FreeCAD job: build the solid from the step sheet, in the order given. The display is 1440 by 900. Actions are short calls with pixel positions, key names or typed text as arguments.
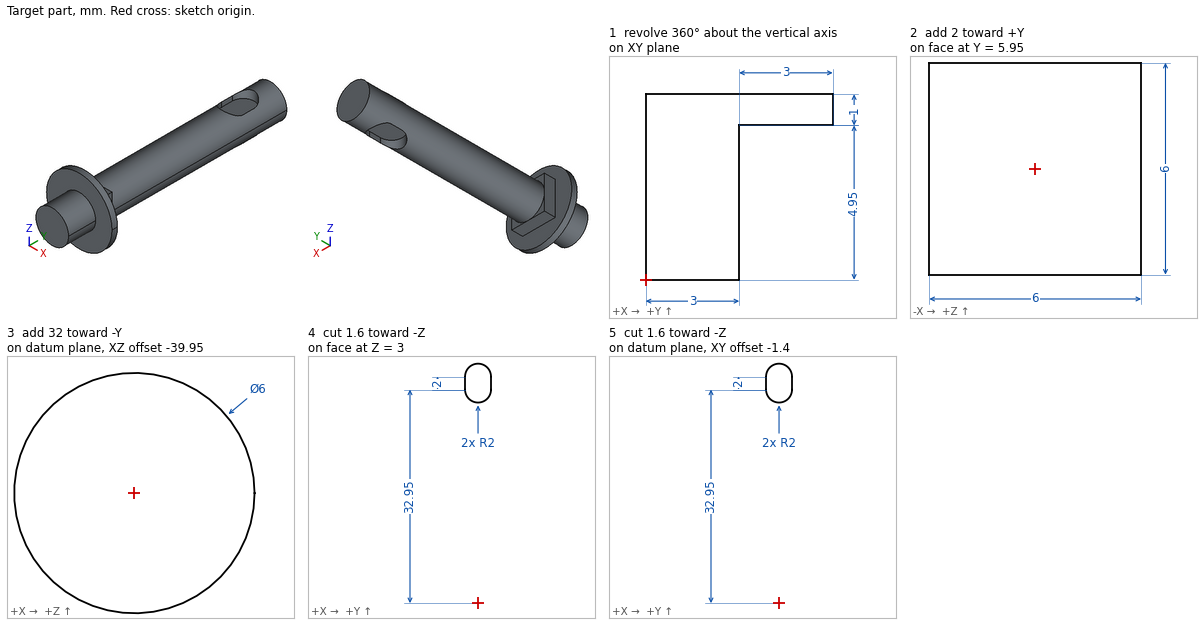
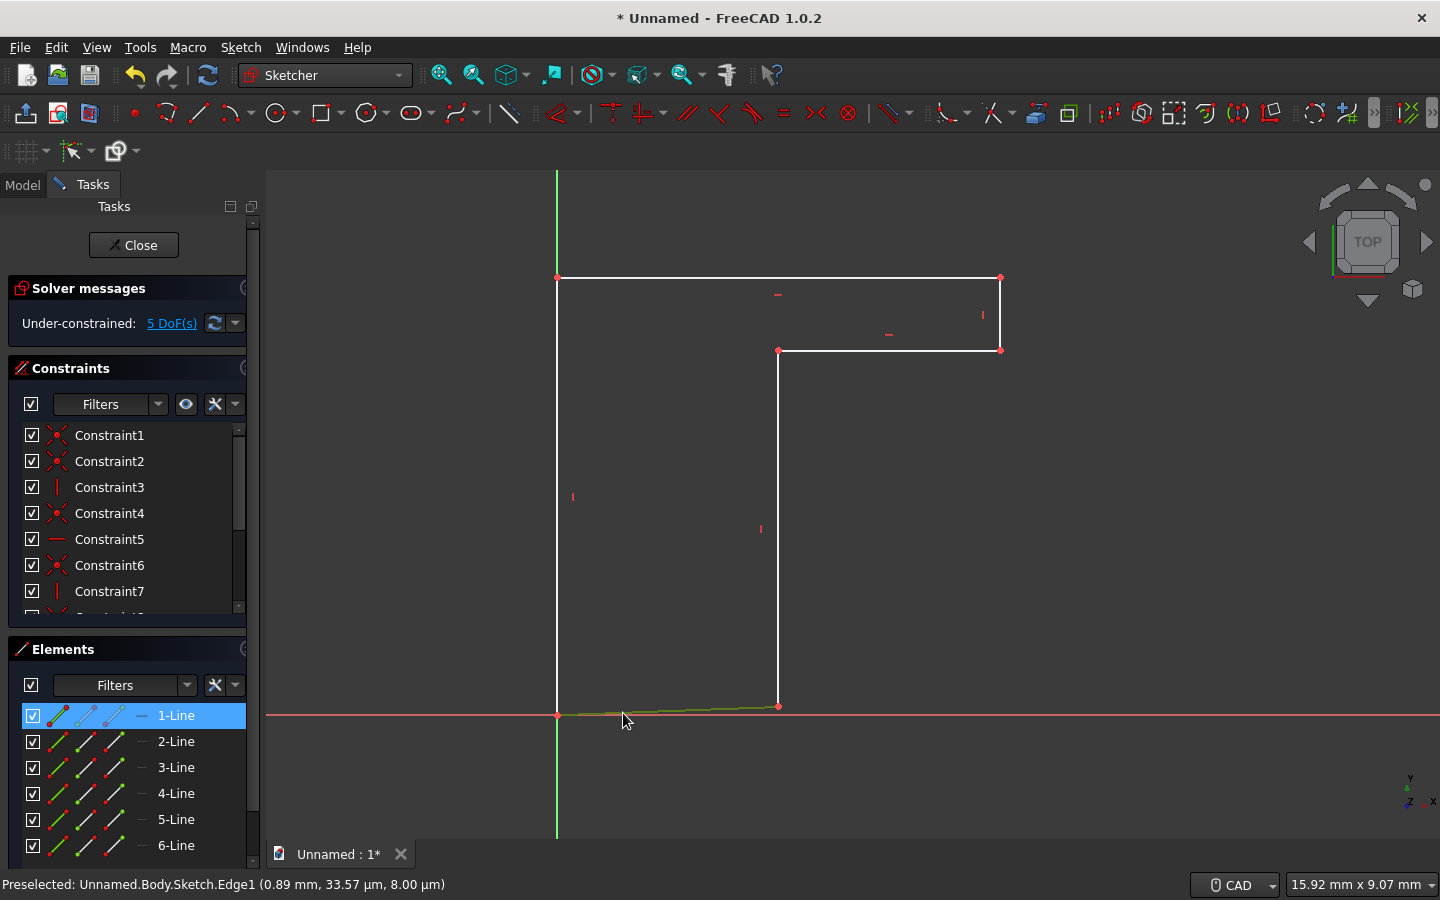
click(666, 114)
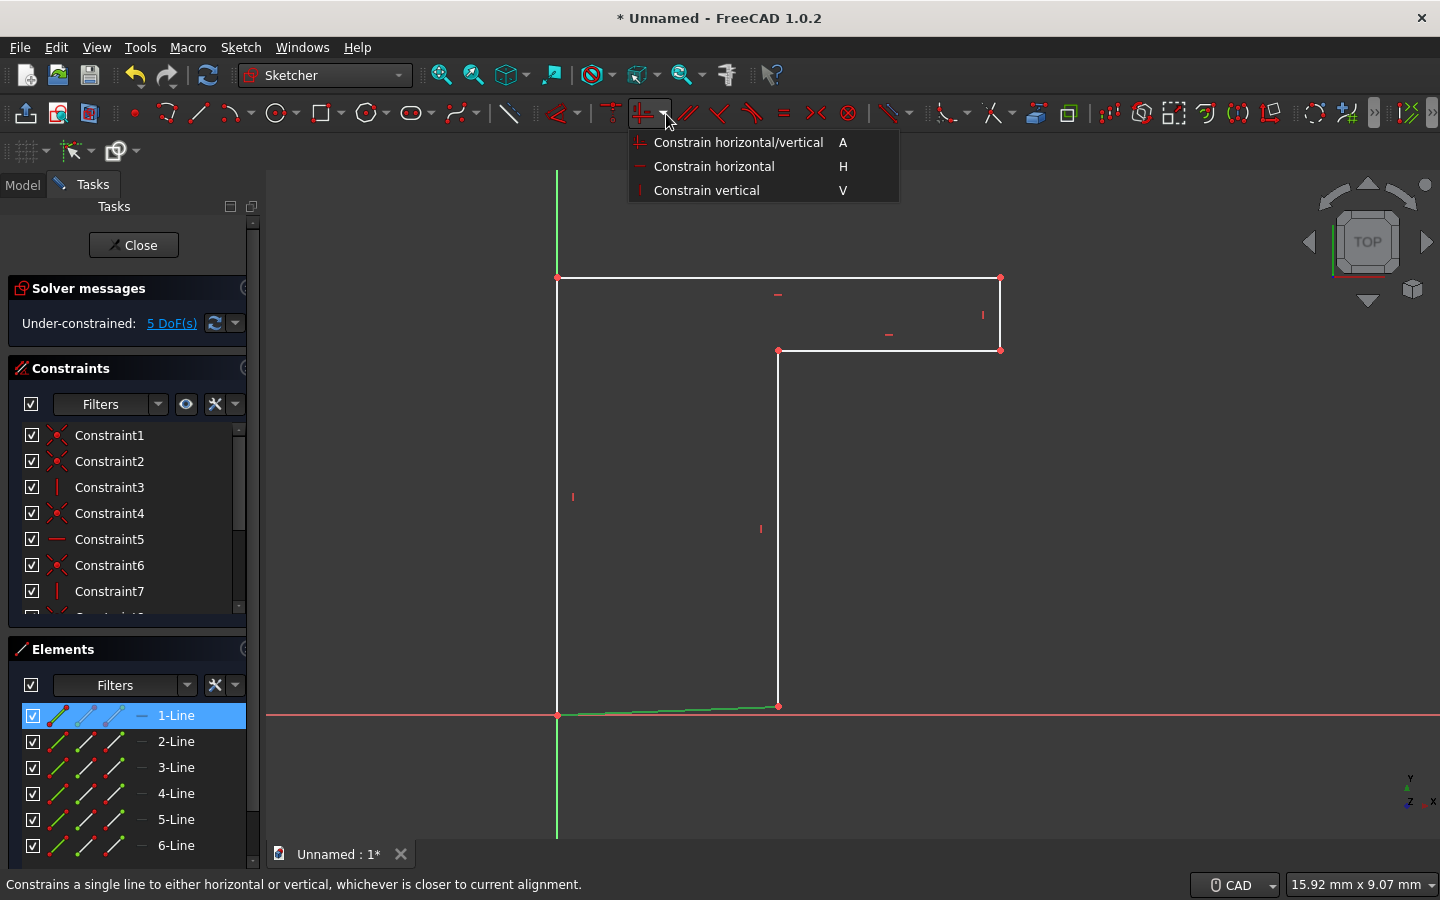
click(764, 166)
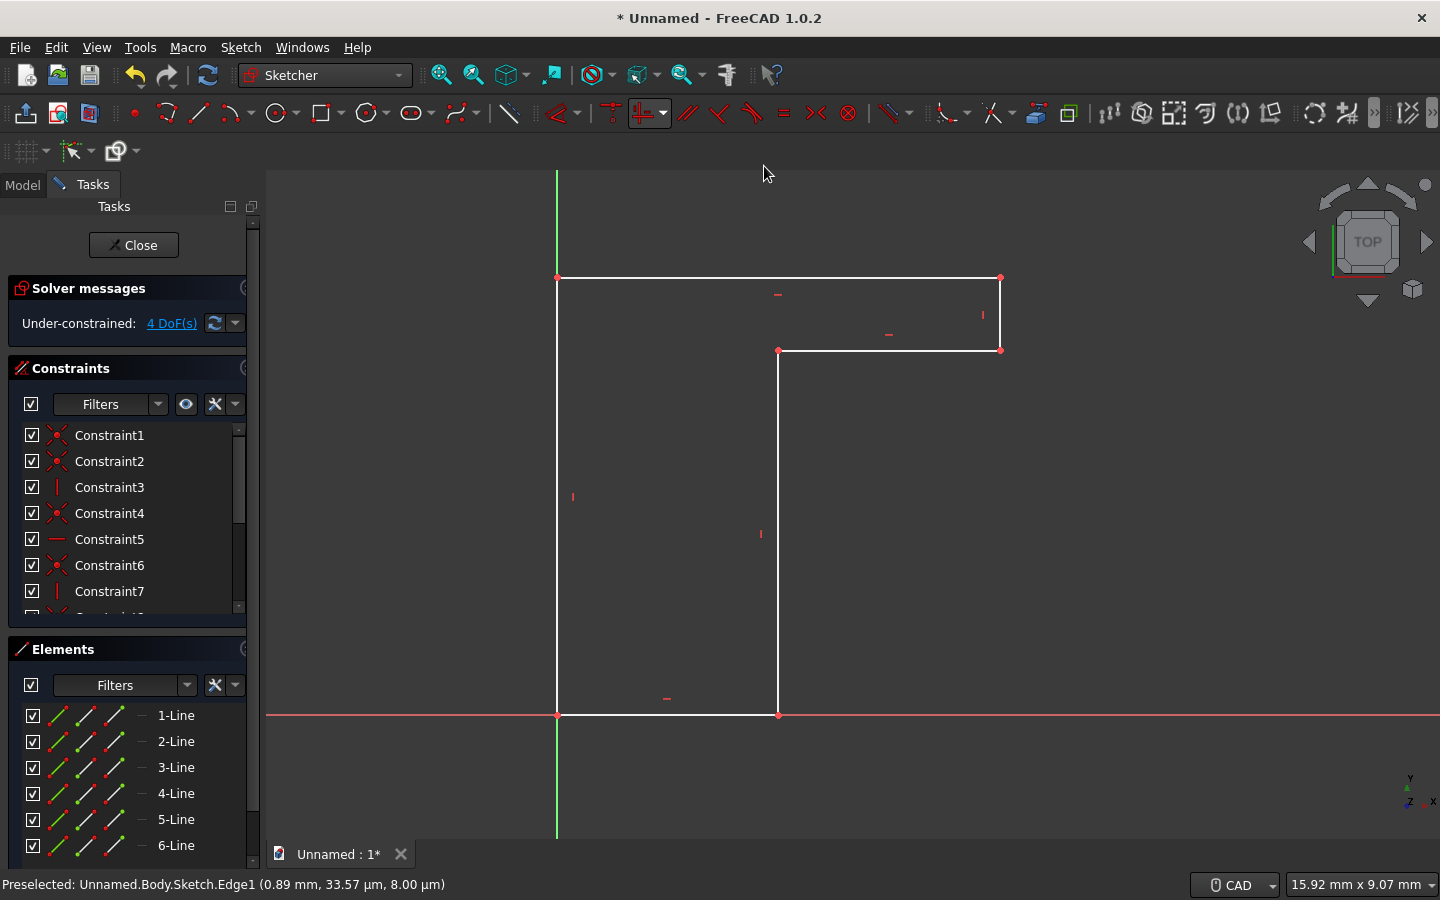
click(623, 715)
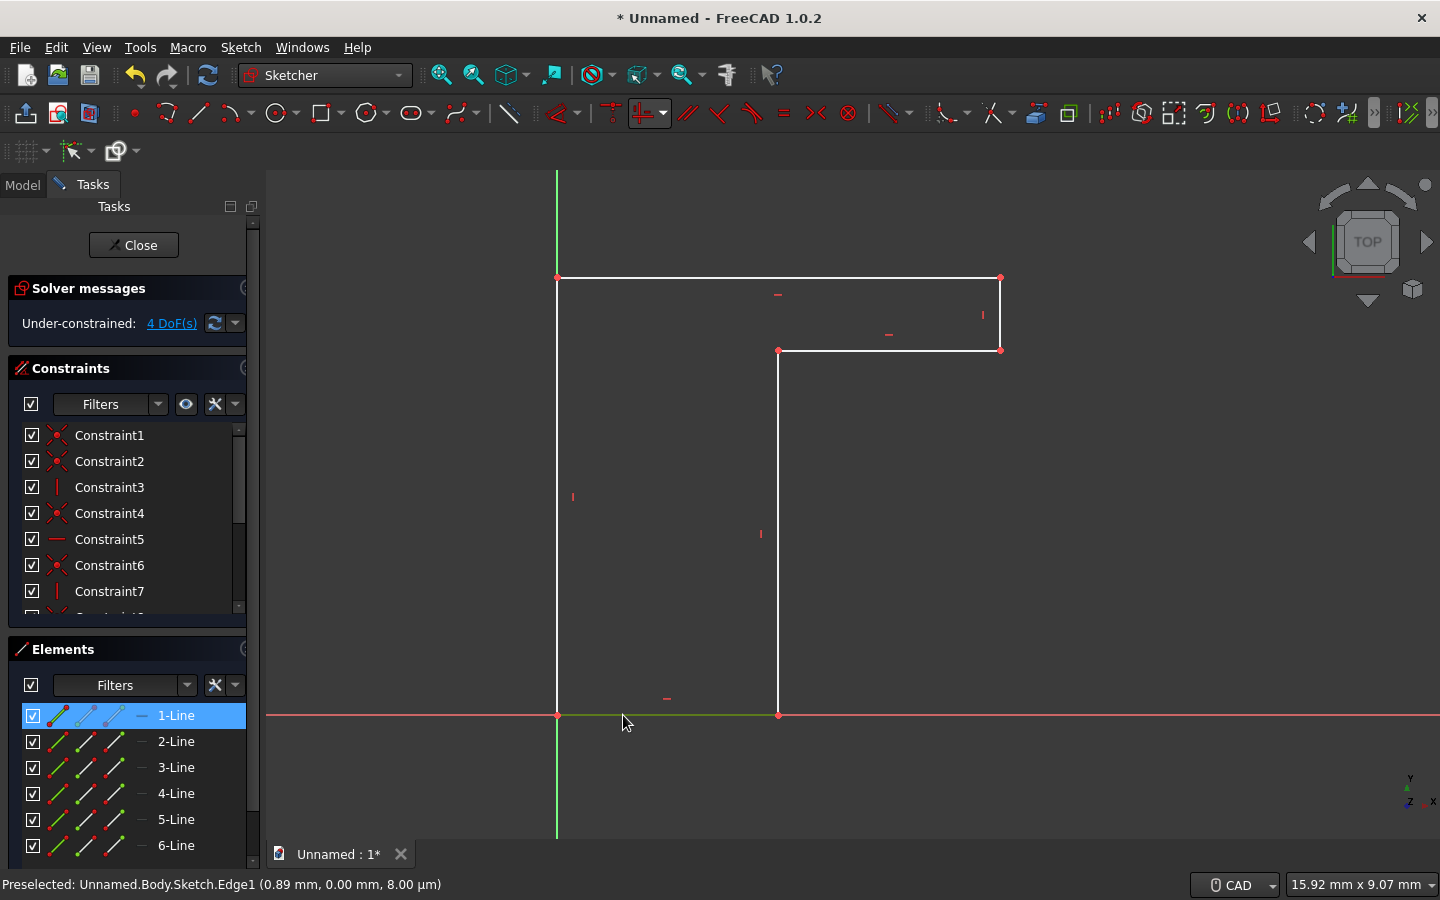
key(l)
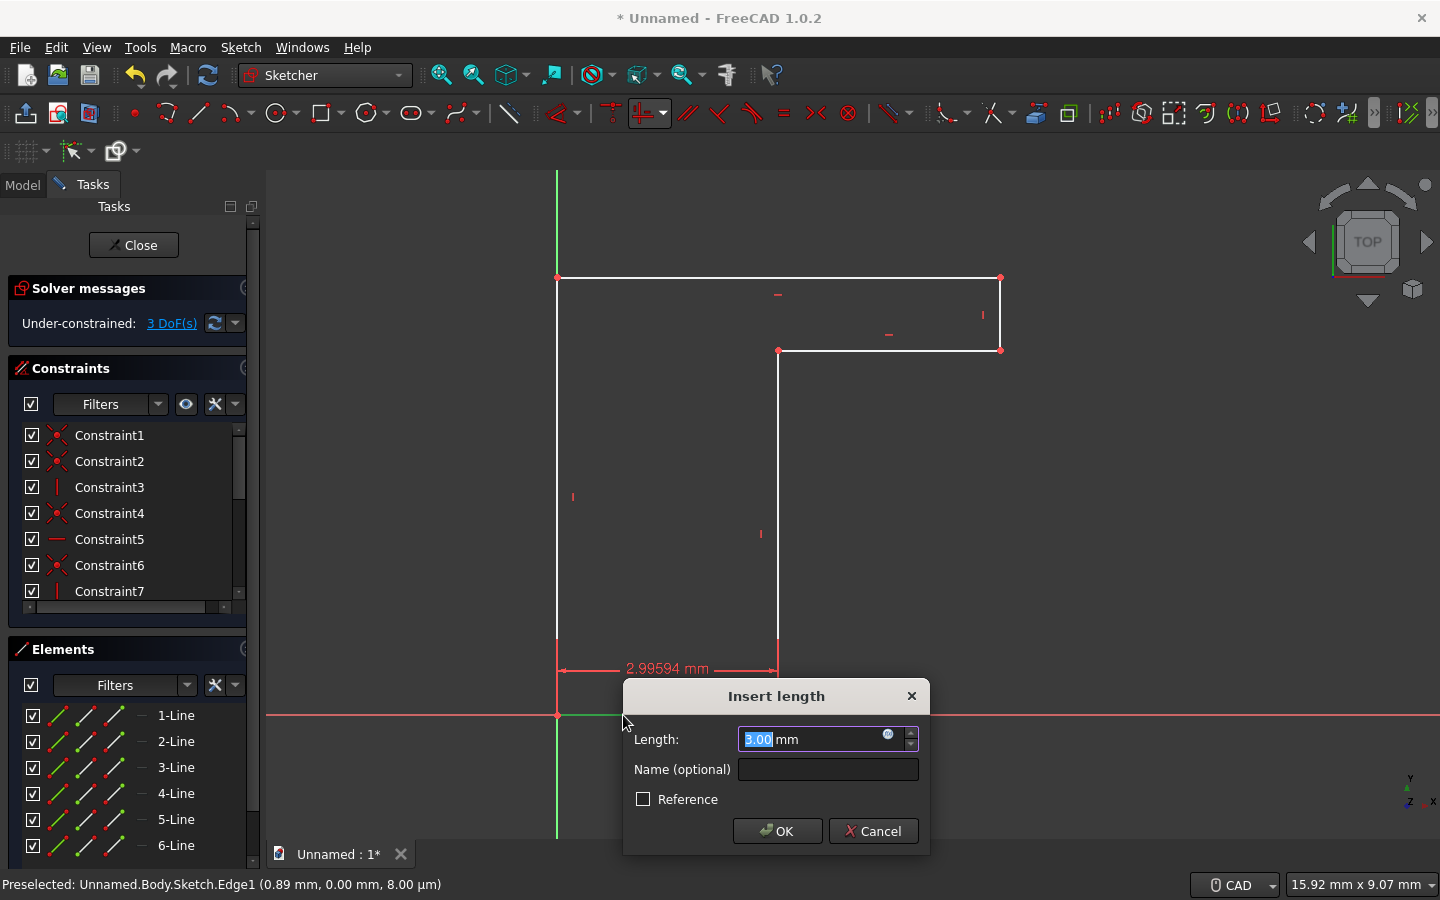
text(3)
key(Return)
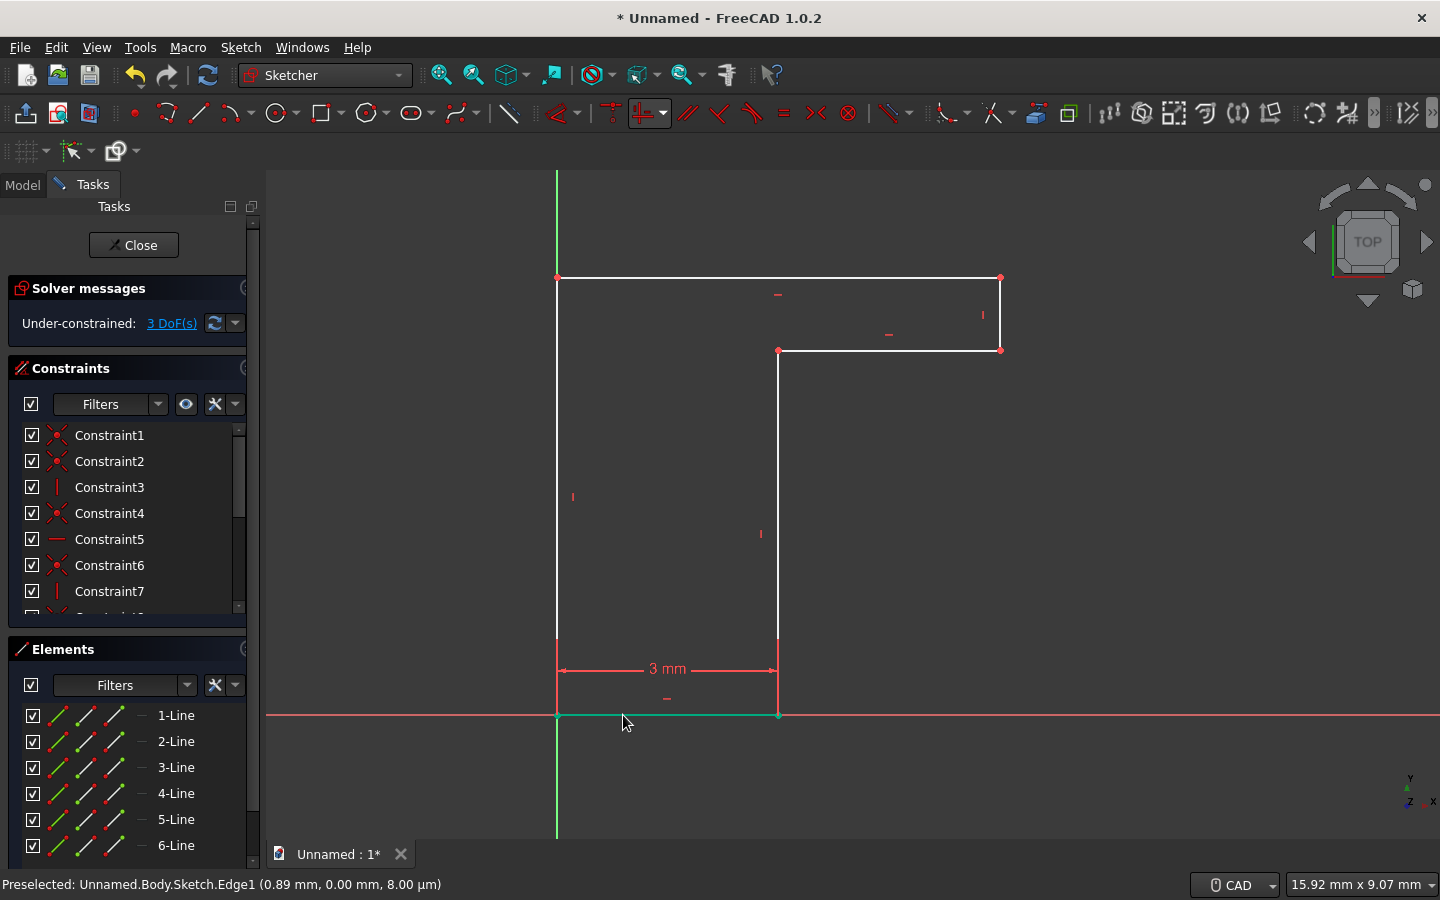
click(845, 351)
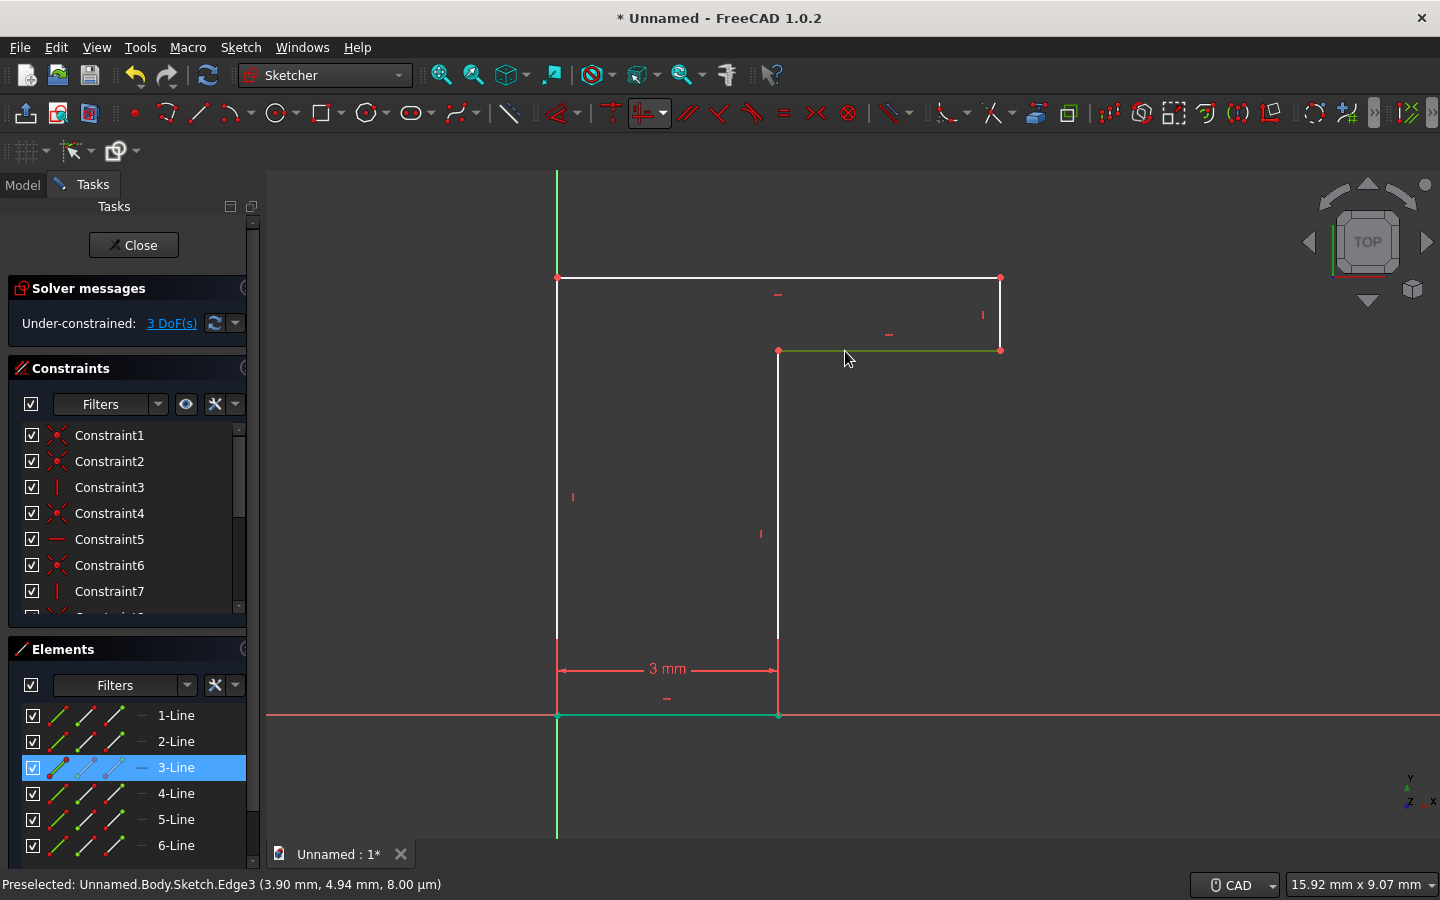
key(l)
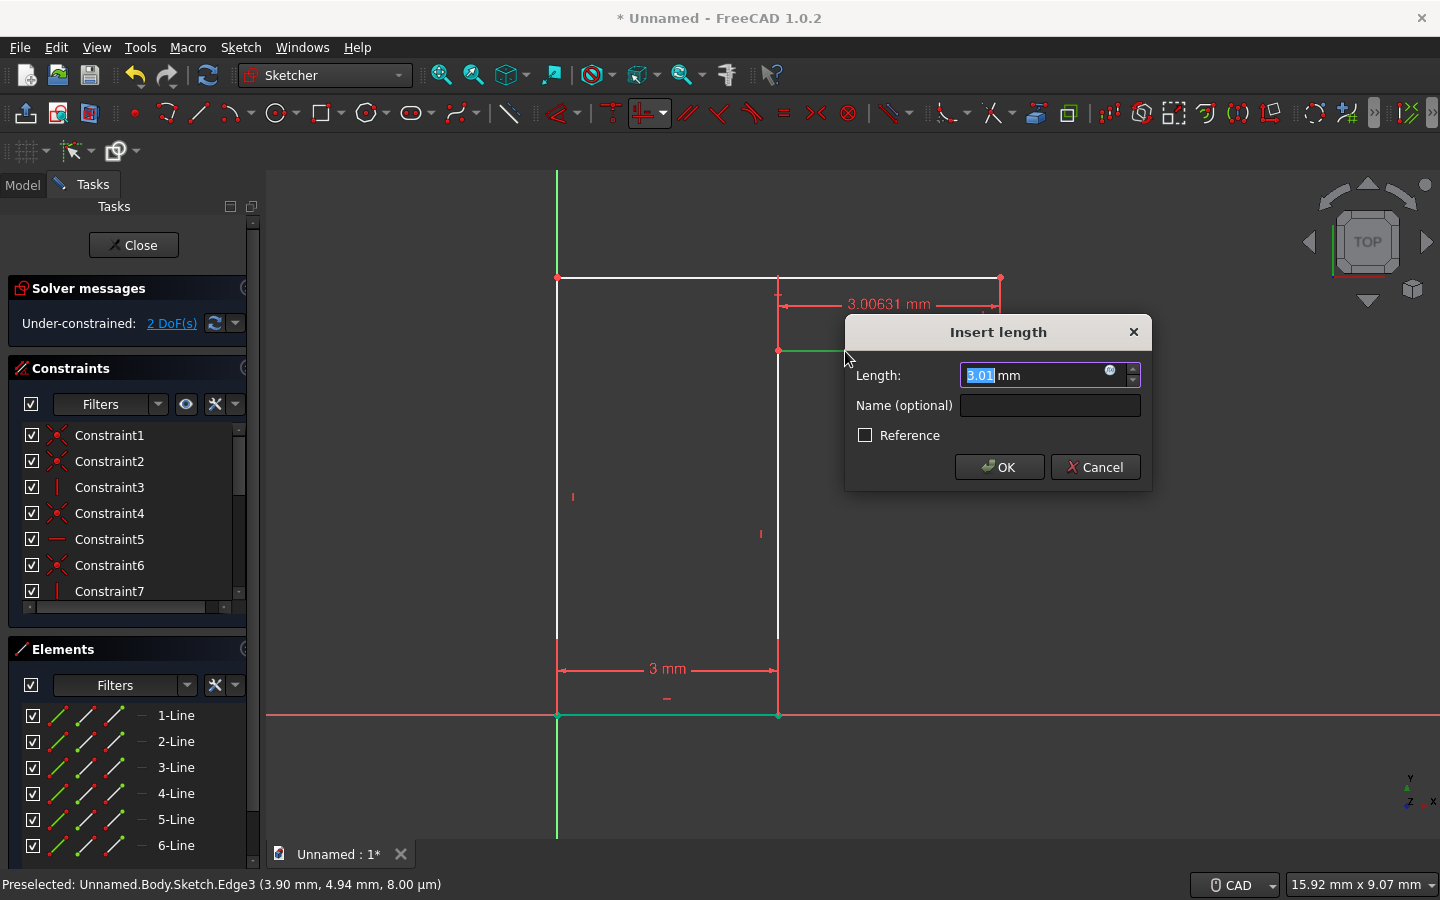
text(3)
key(Return)